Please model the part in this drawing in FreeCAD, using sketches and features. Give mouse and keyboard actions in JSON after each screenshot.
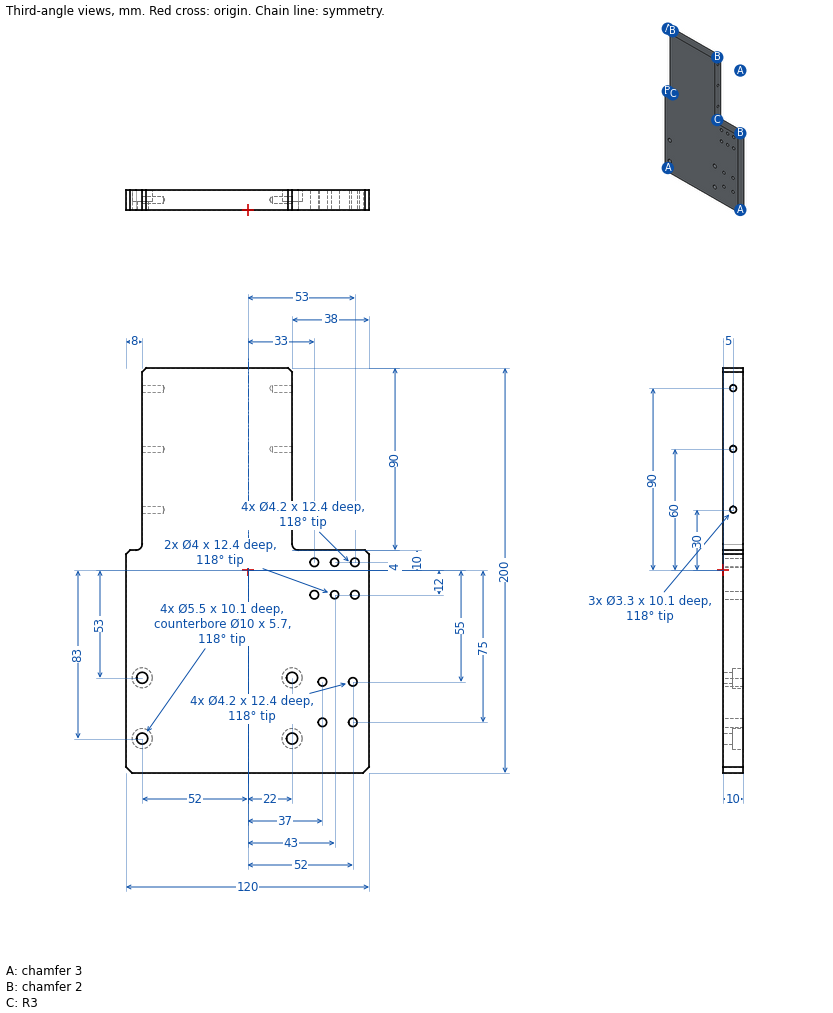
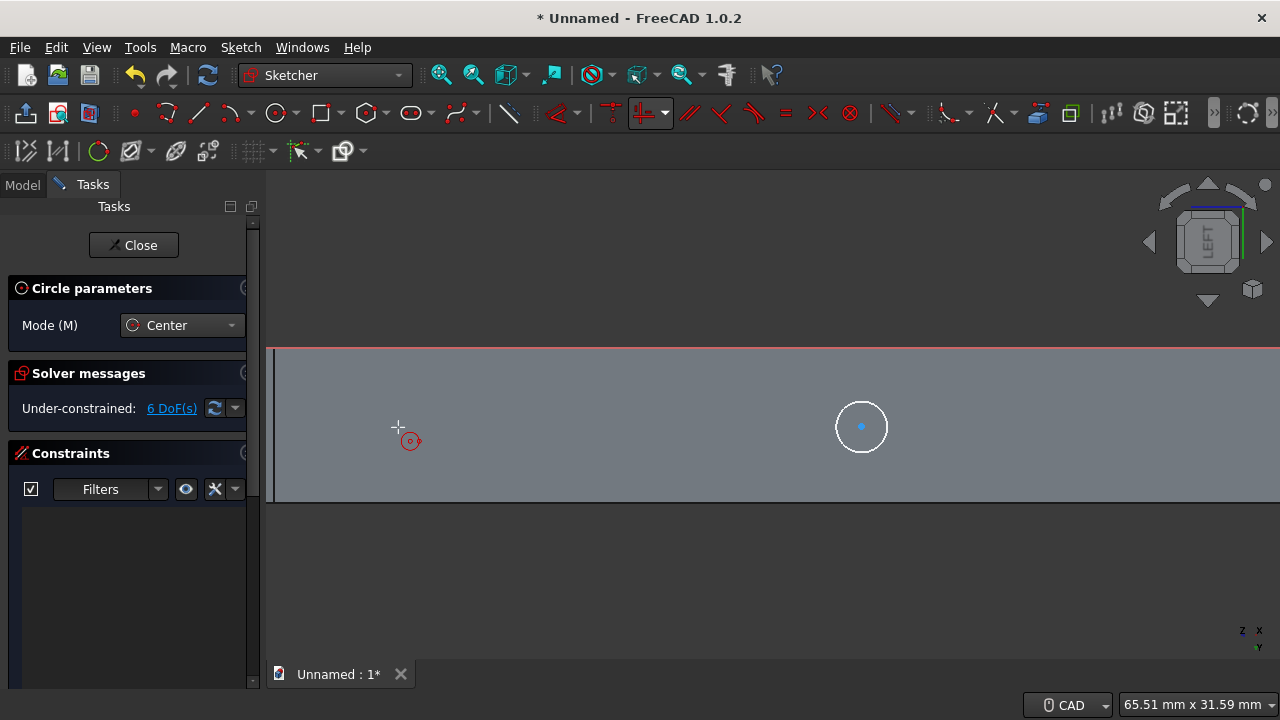
{"action": "left_click", "coordinate": [398, 426]}
{"action": "left_click", "coordinate": [416, 408]}
{"action": "key", "text": "Escape"}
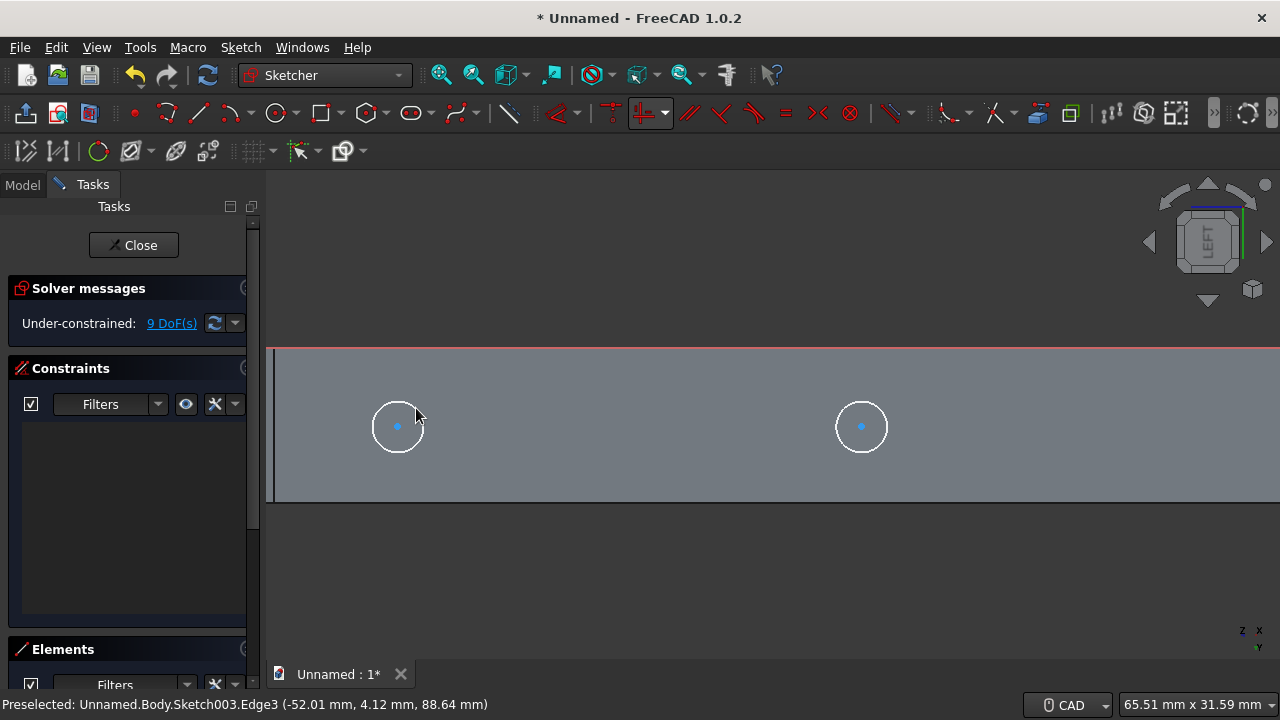
{"action": "scroll", "coordinate": [397, 427], "scroll_direction": "down", "scroll_amount": 4}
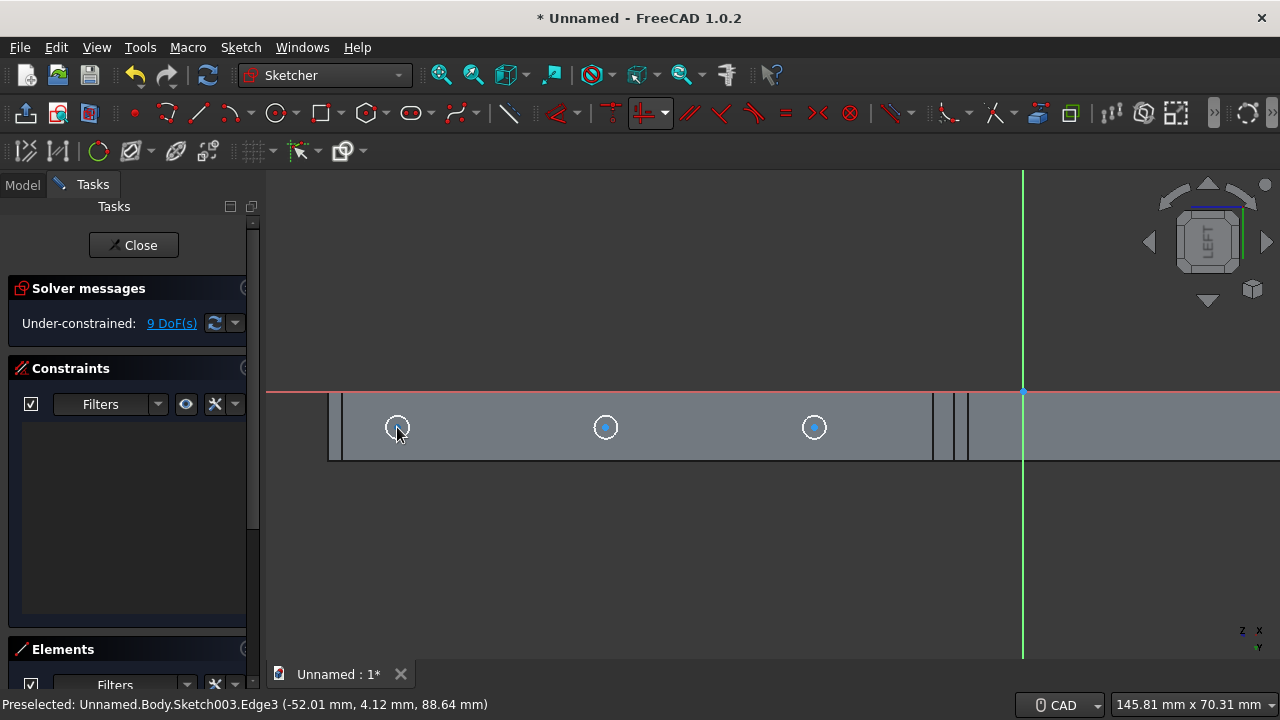
{"action": "left_click", "coordinate": [822, 419]}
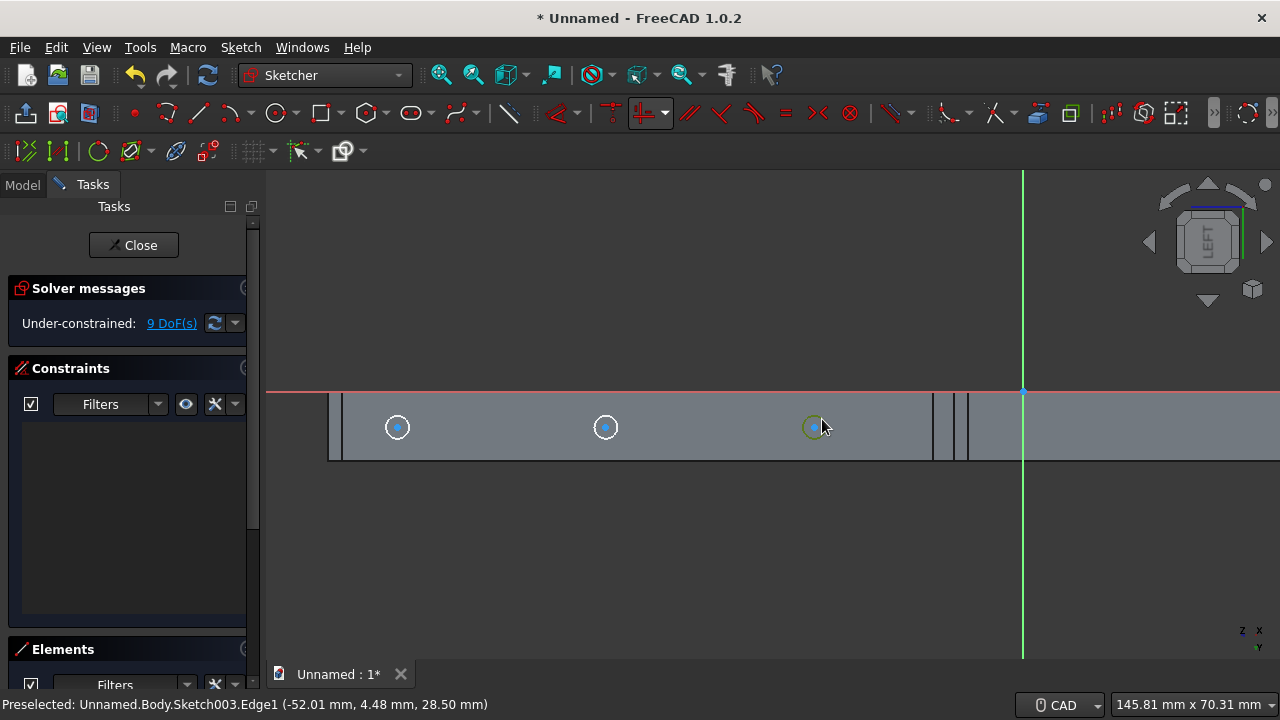
{"action": "left_click", "coordinate": [614, 419]}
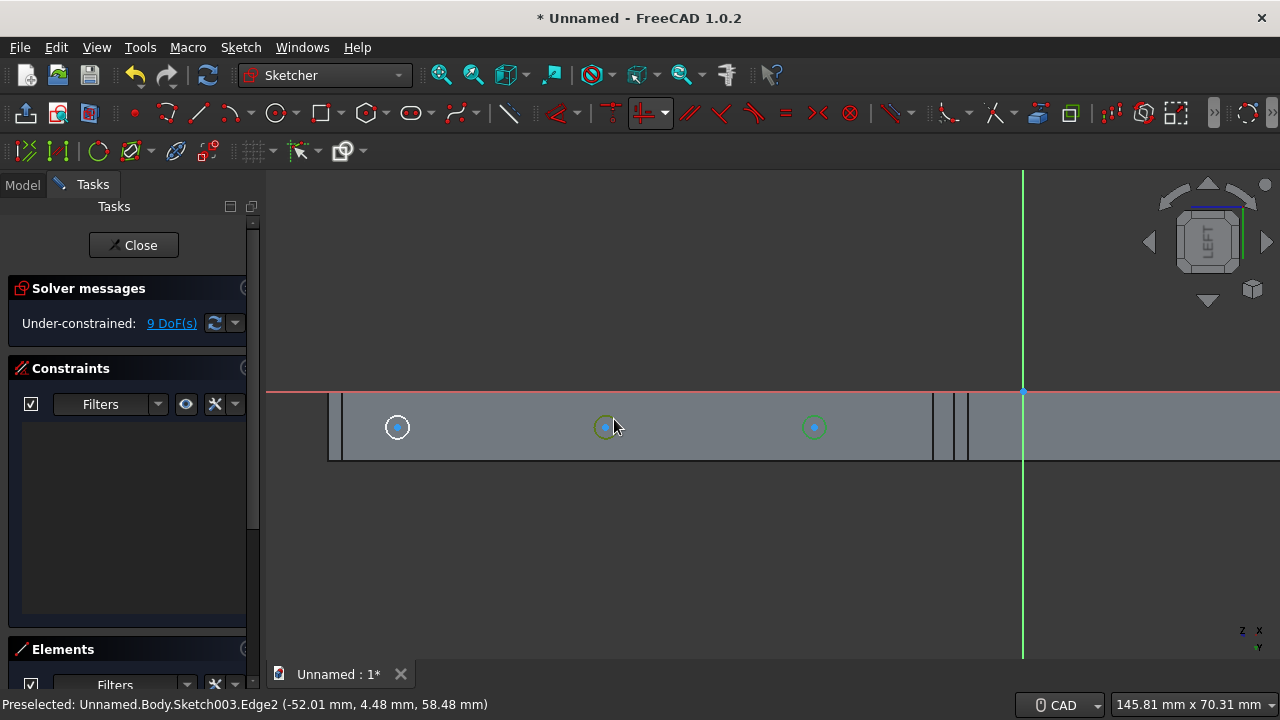
{"action": "left_click", "coordinate": [406, 419]}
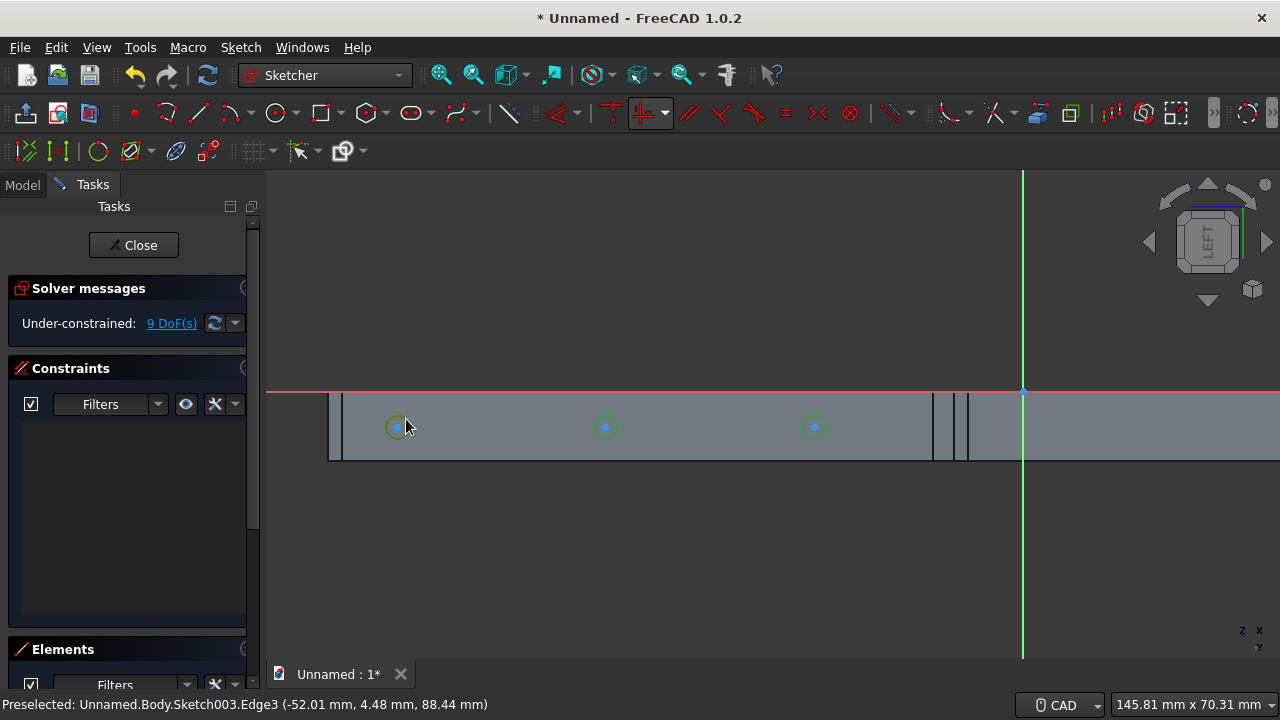
{"action": "left_click", "coordinate": [786, 114]}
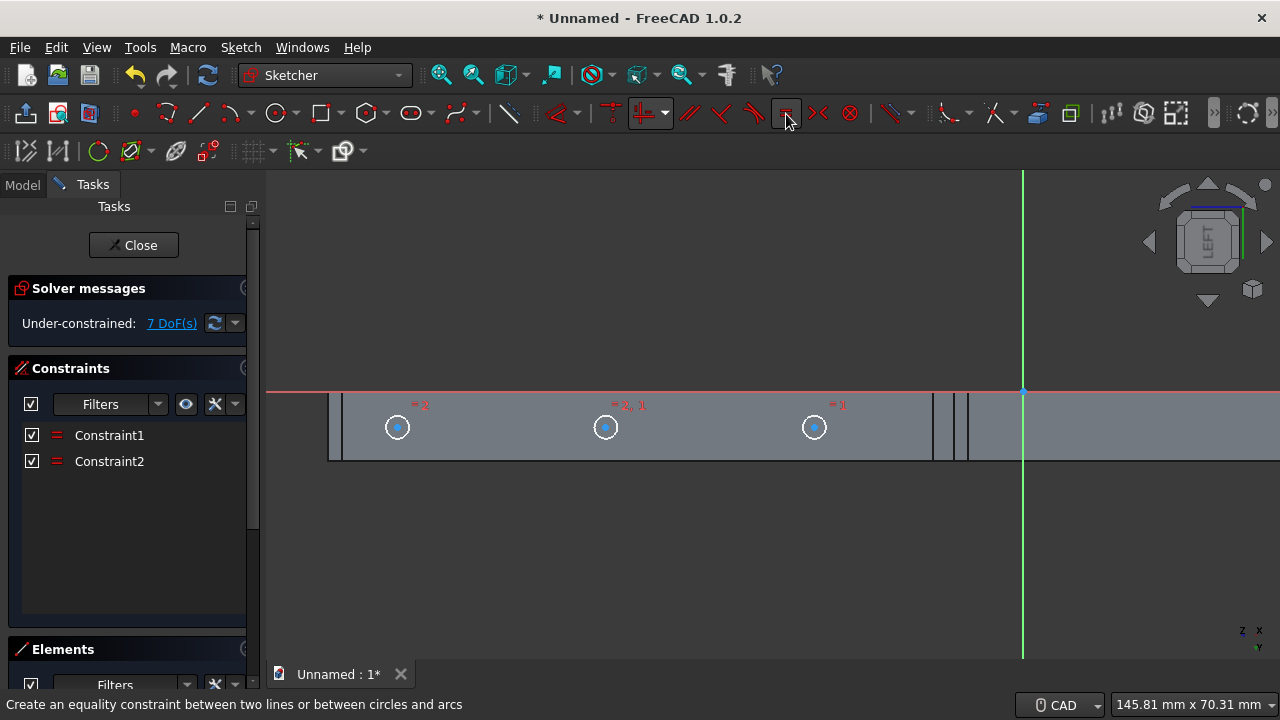
{"action": "left_click", "coordinate": [814, 427]}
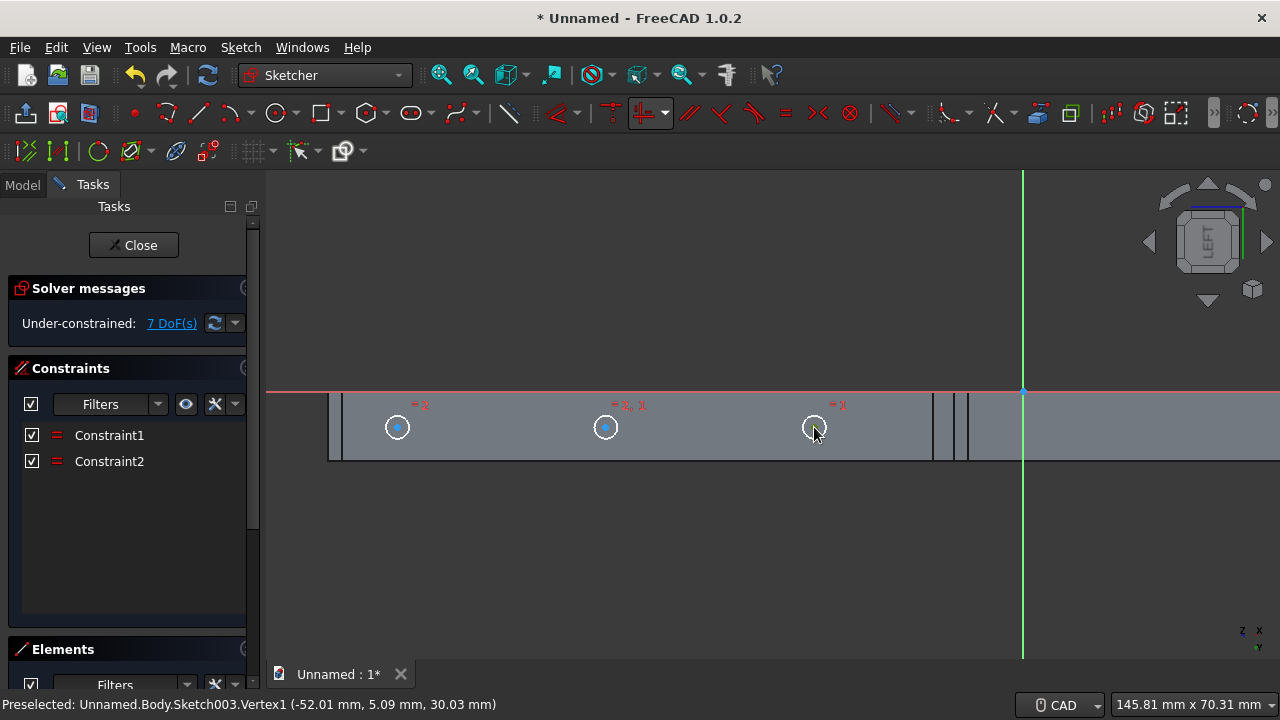
{"action": "left_click", "coordinate": [606, 427]}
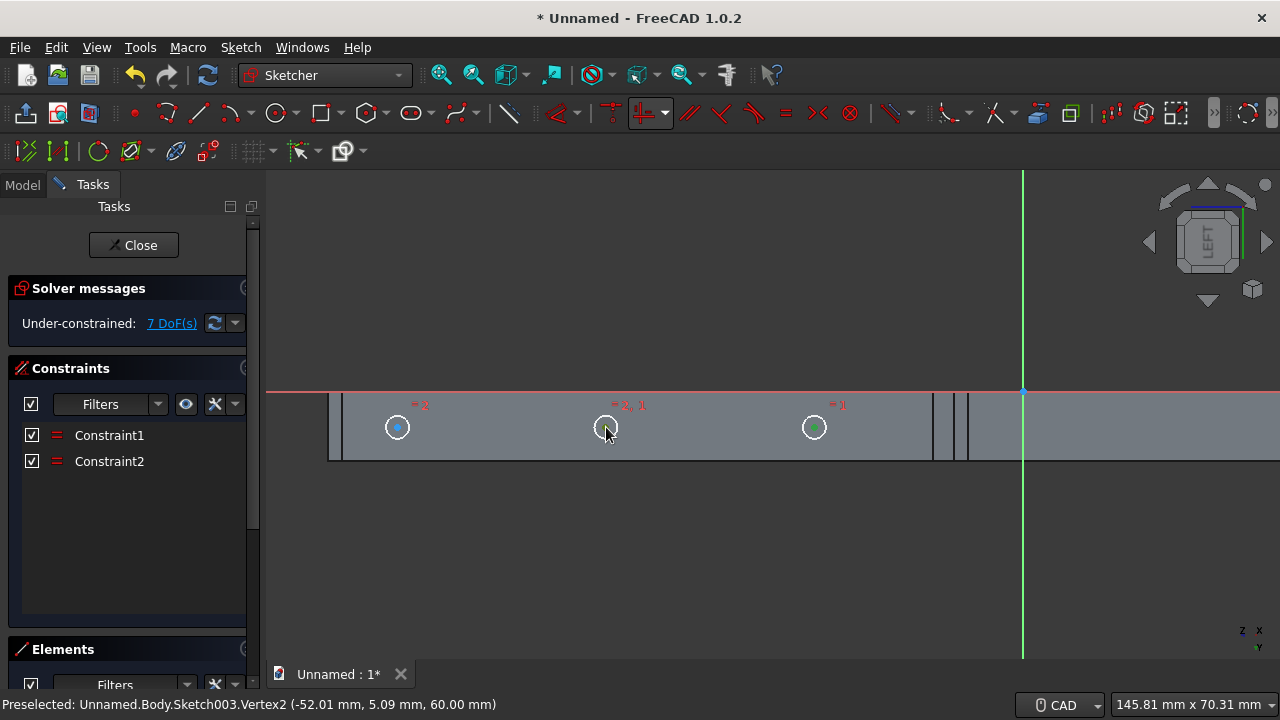
{"action": "key", "text": "h"}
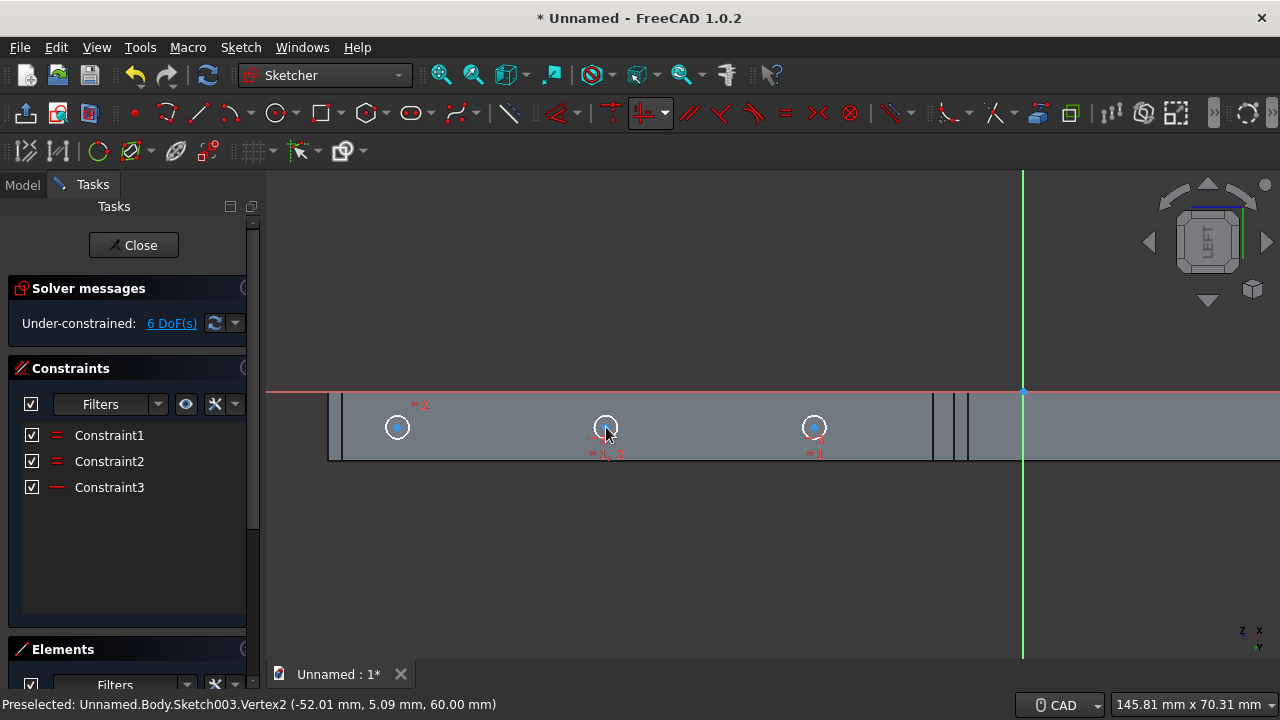
{"action": "left_click", "coordinate": [606, 427]}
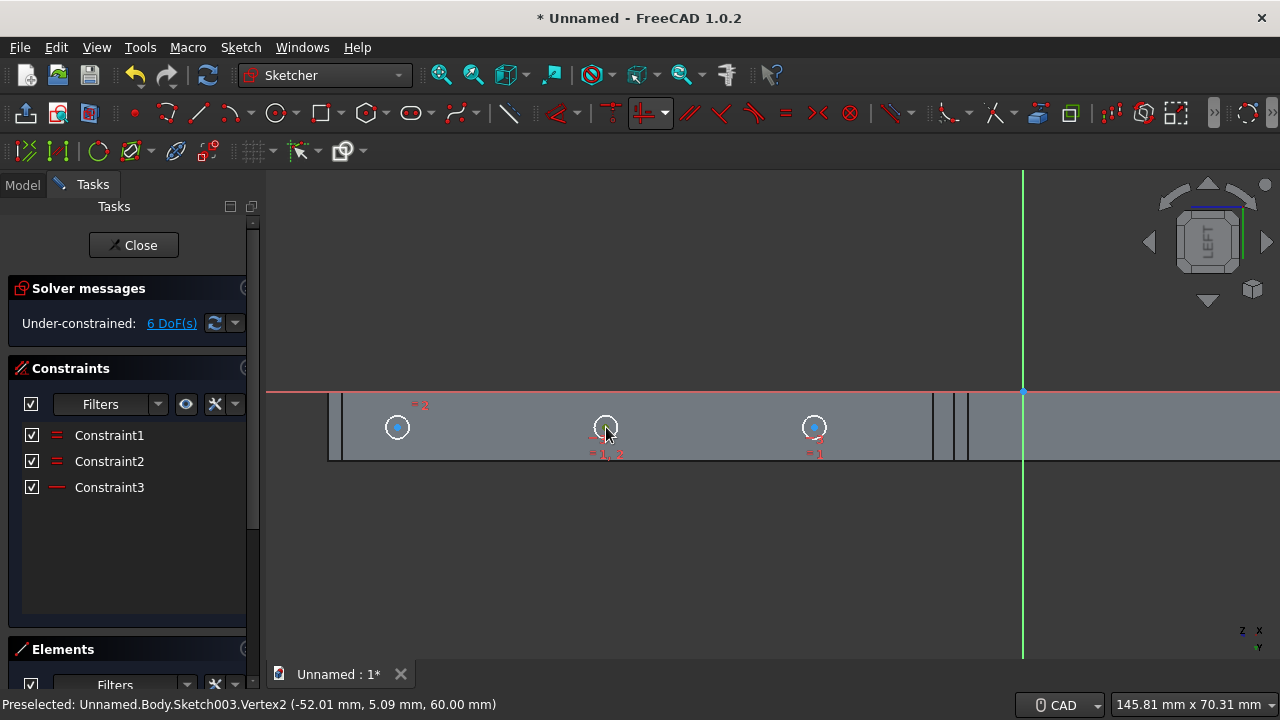
{"action": "left_click", "coordinate": [398, 427]}